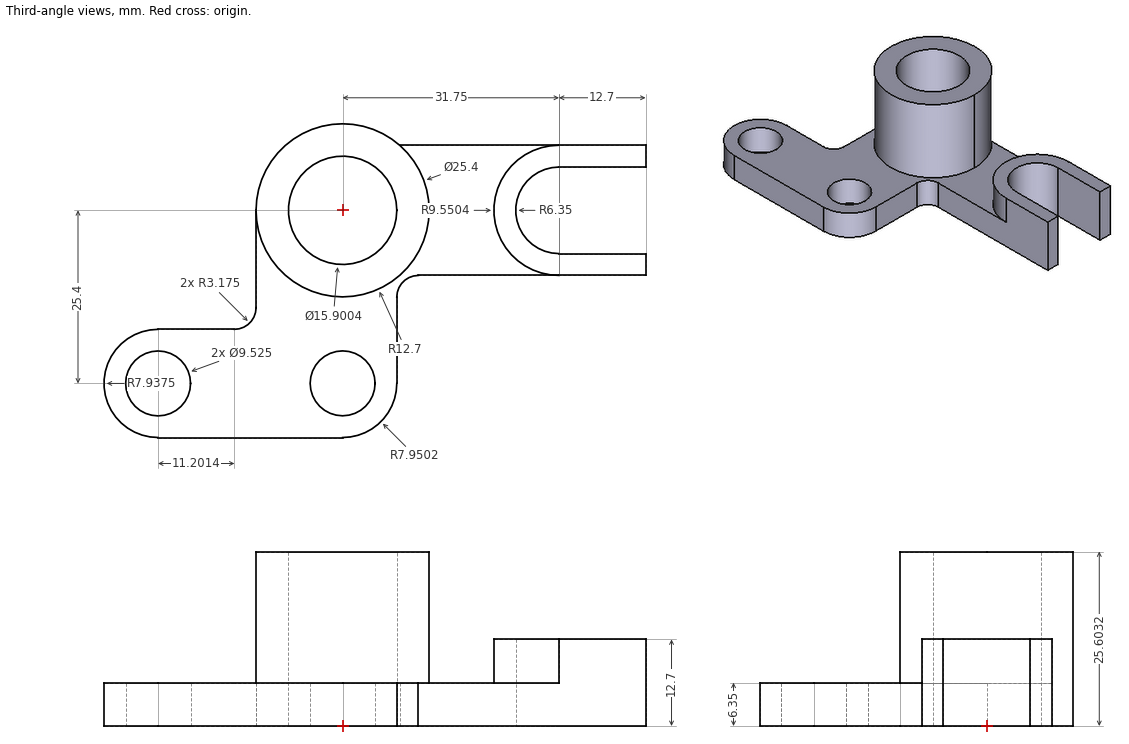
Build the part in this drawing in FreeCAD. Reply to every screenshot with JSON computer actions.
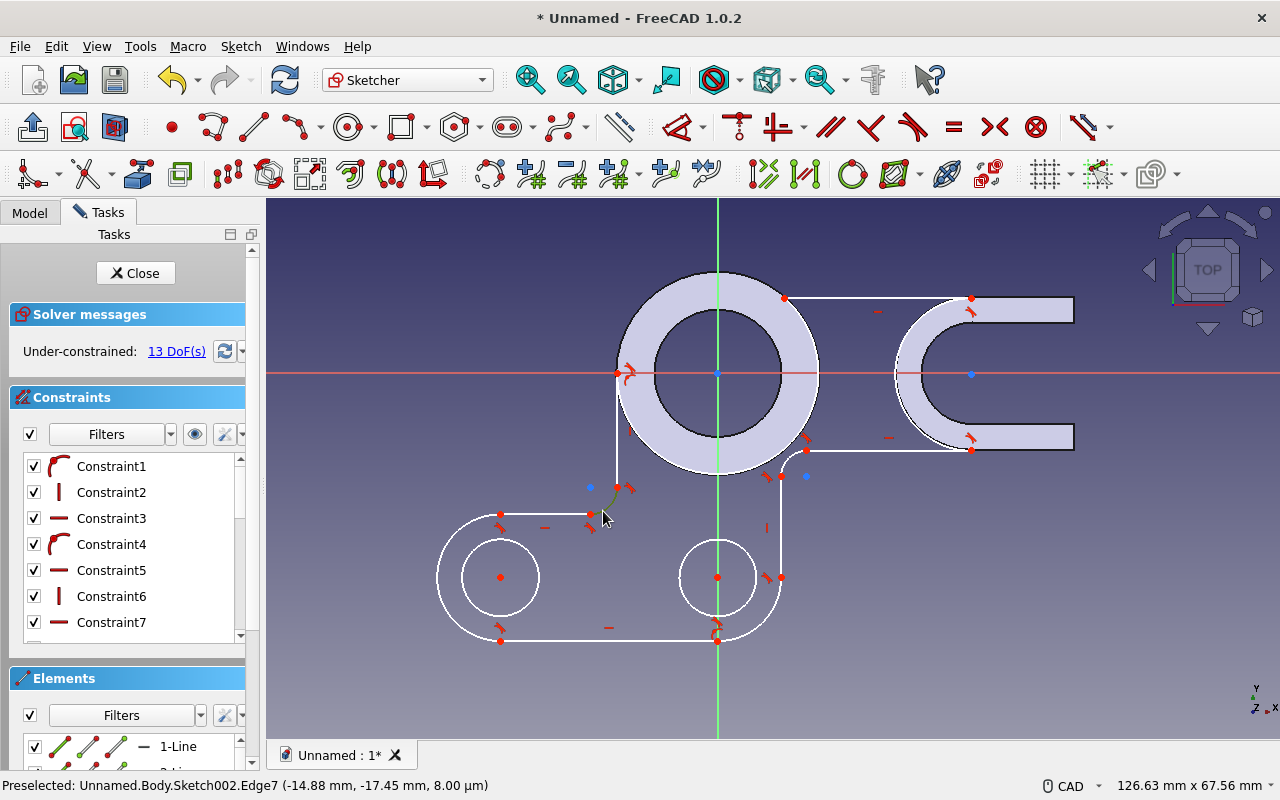
{"action": "scroll", "coordinate": [795, 454], "scroll_direction": "up", "scroll_amount": 2}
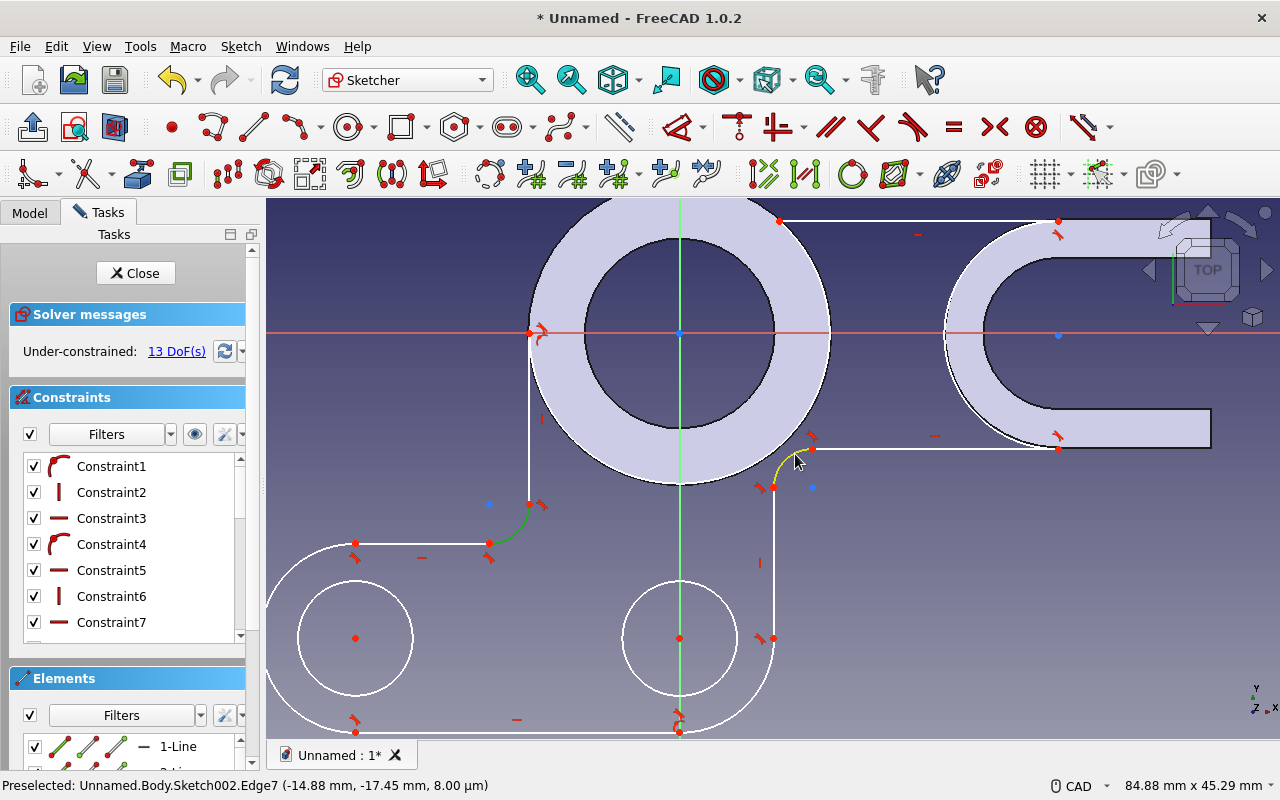
{"action": "left_click", "coordinate": [795, 453]}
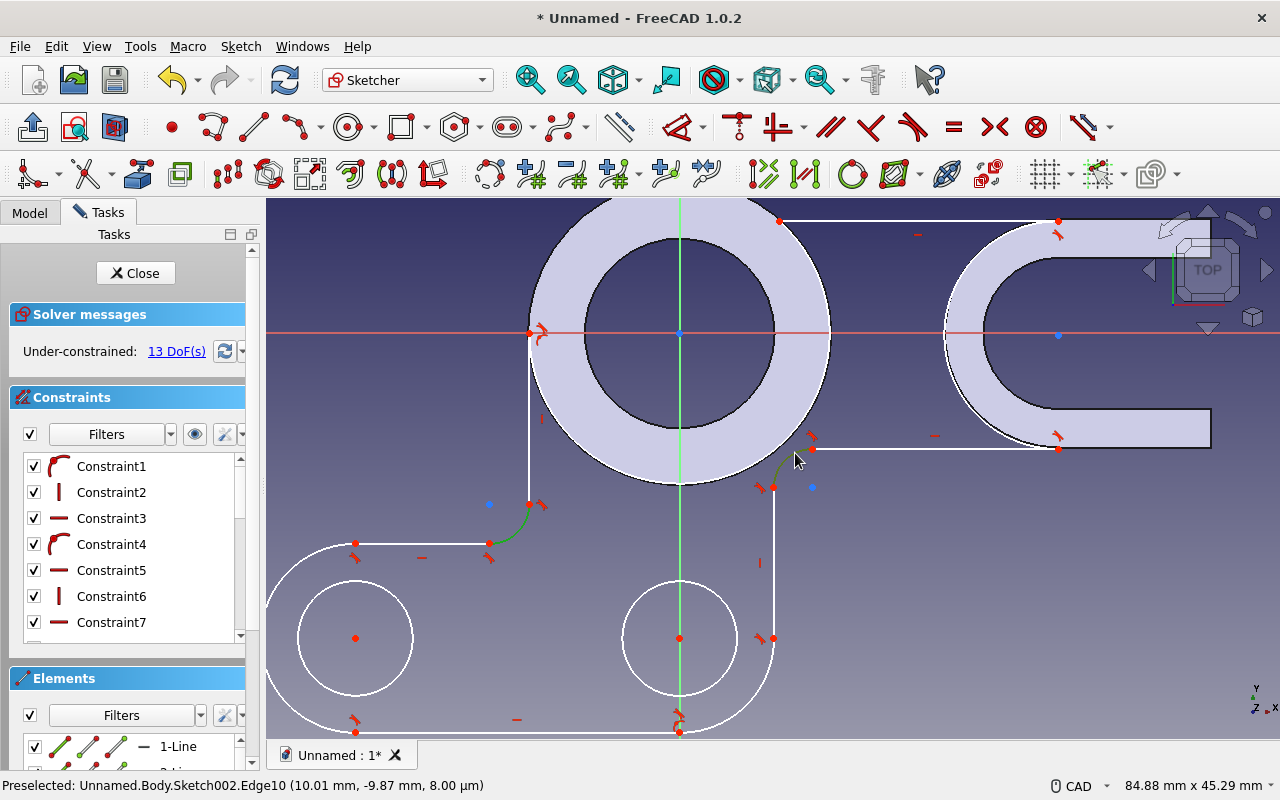
{"action": "left_click", "coordinate": [954, 128]}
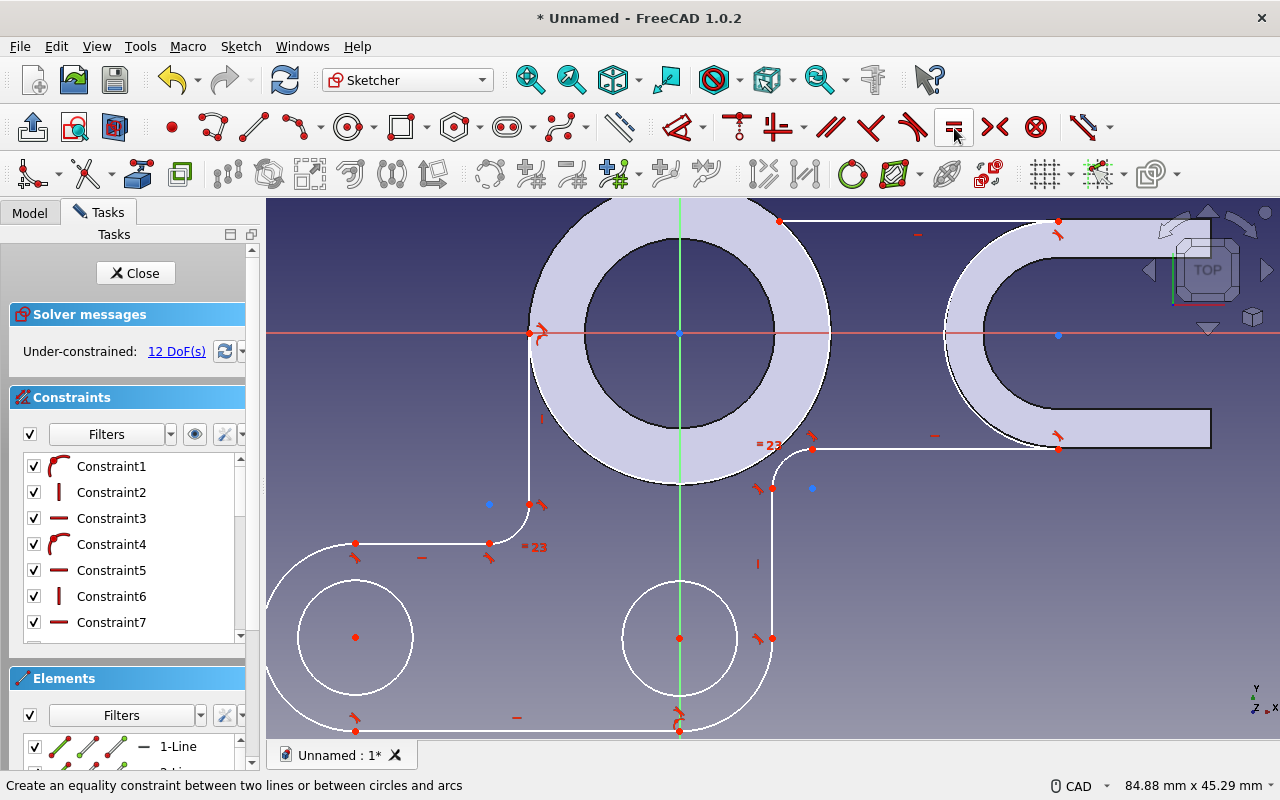
{"action": "left_click", "coordinate": [396, 597]}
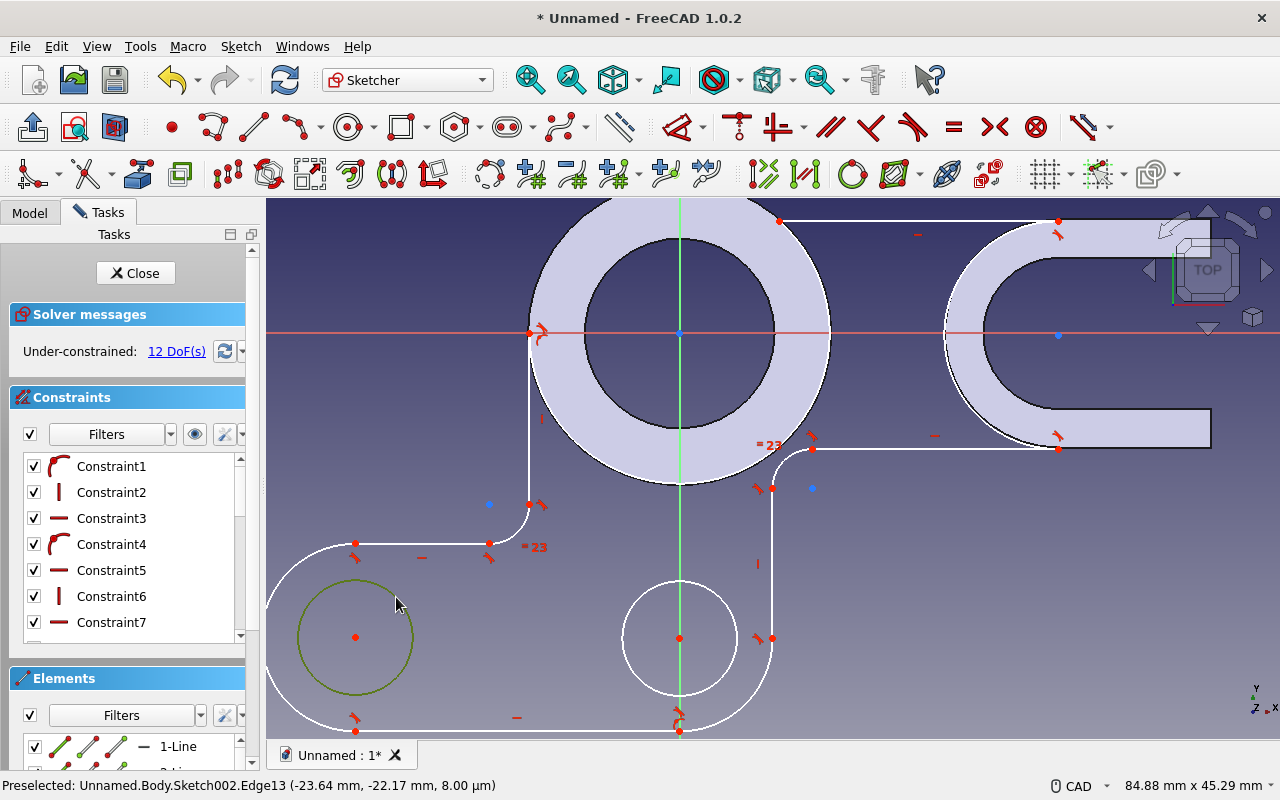
{"action": "left_click", "coordinate": [720, 598]}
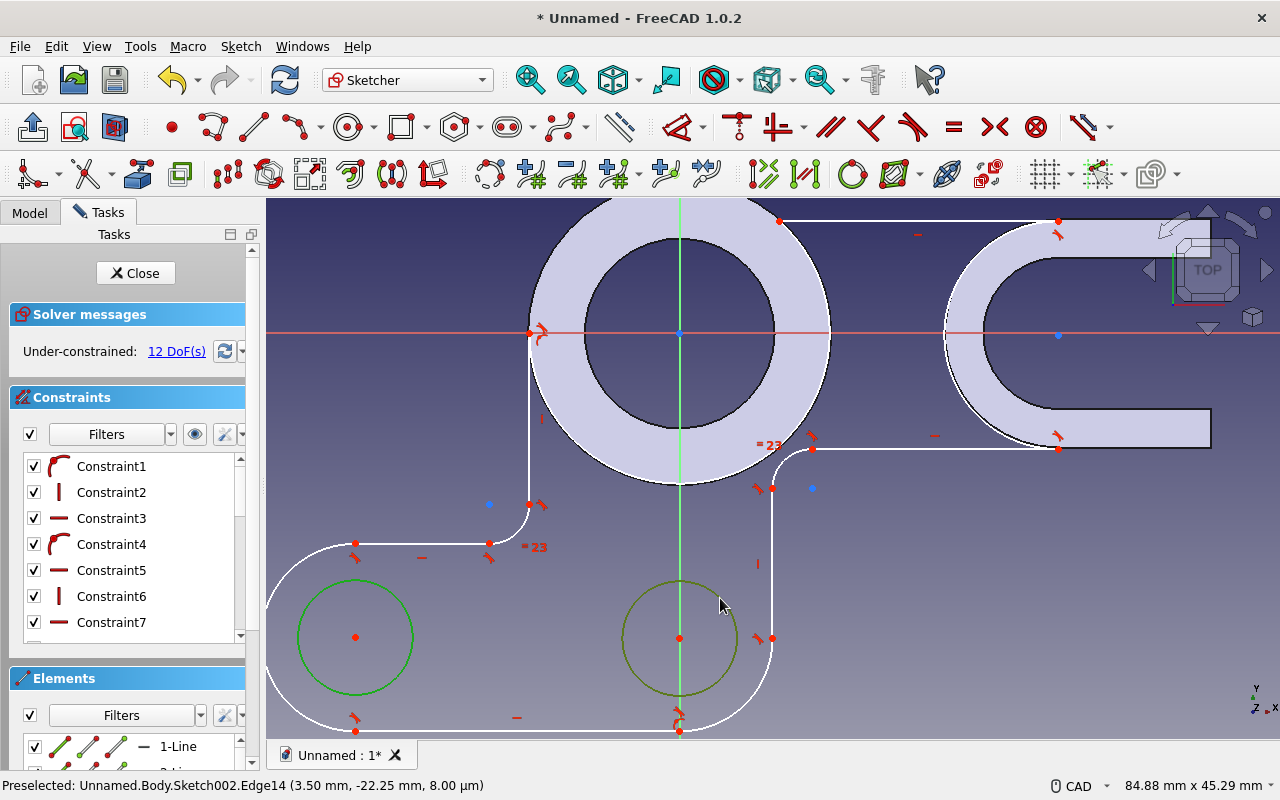
{"action": "left_click", "coordinate": [954, 128]}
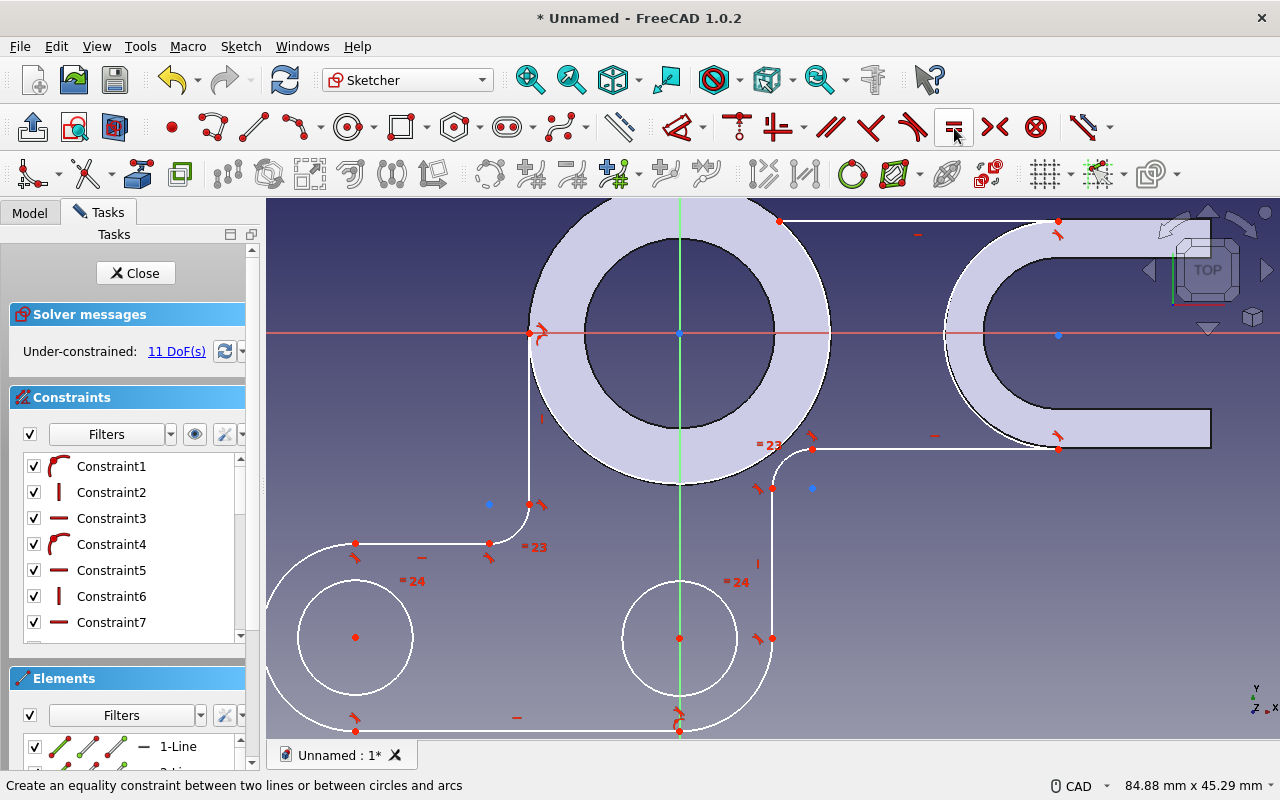
{"action": "left_click", "coordinate": [1058, 335]}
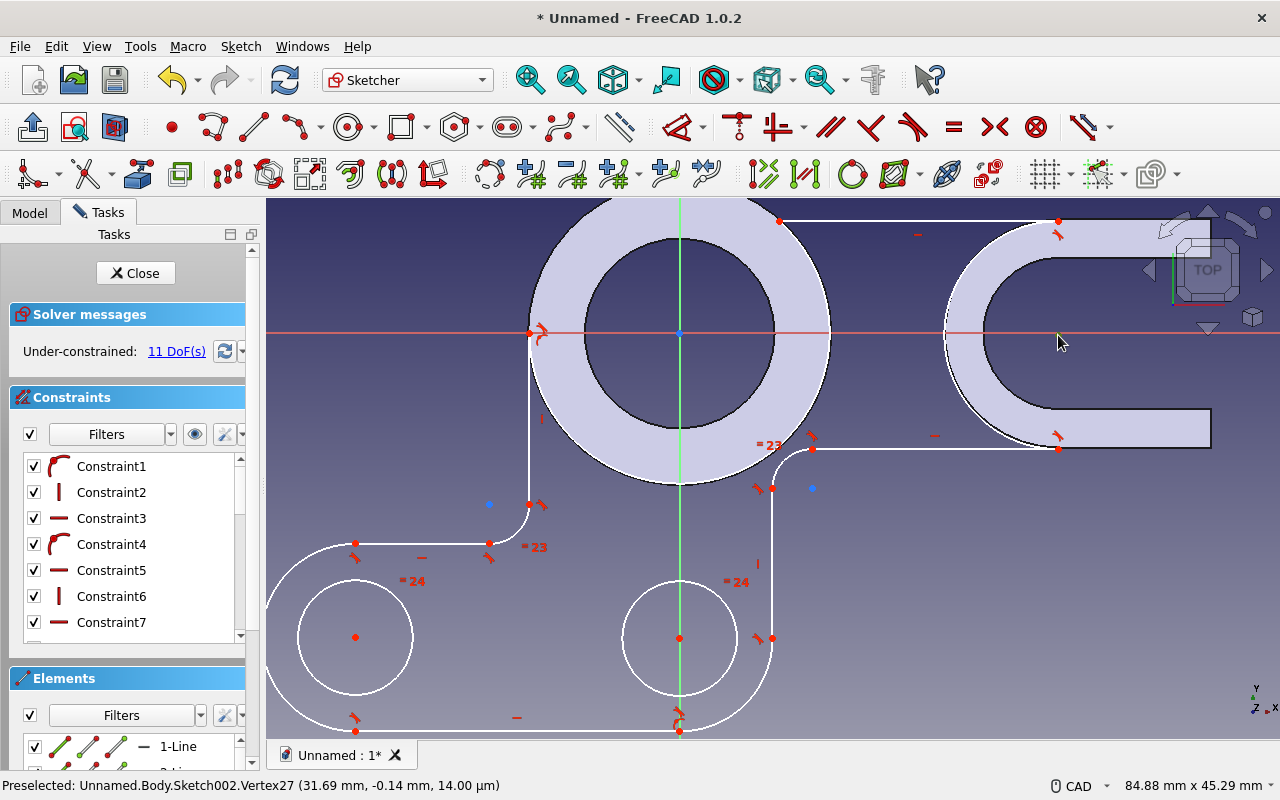
{"action": "left_click", "coordinate": [353, 333]}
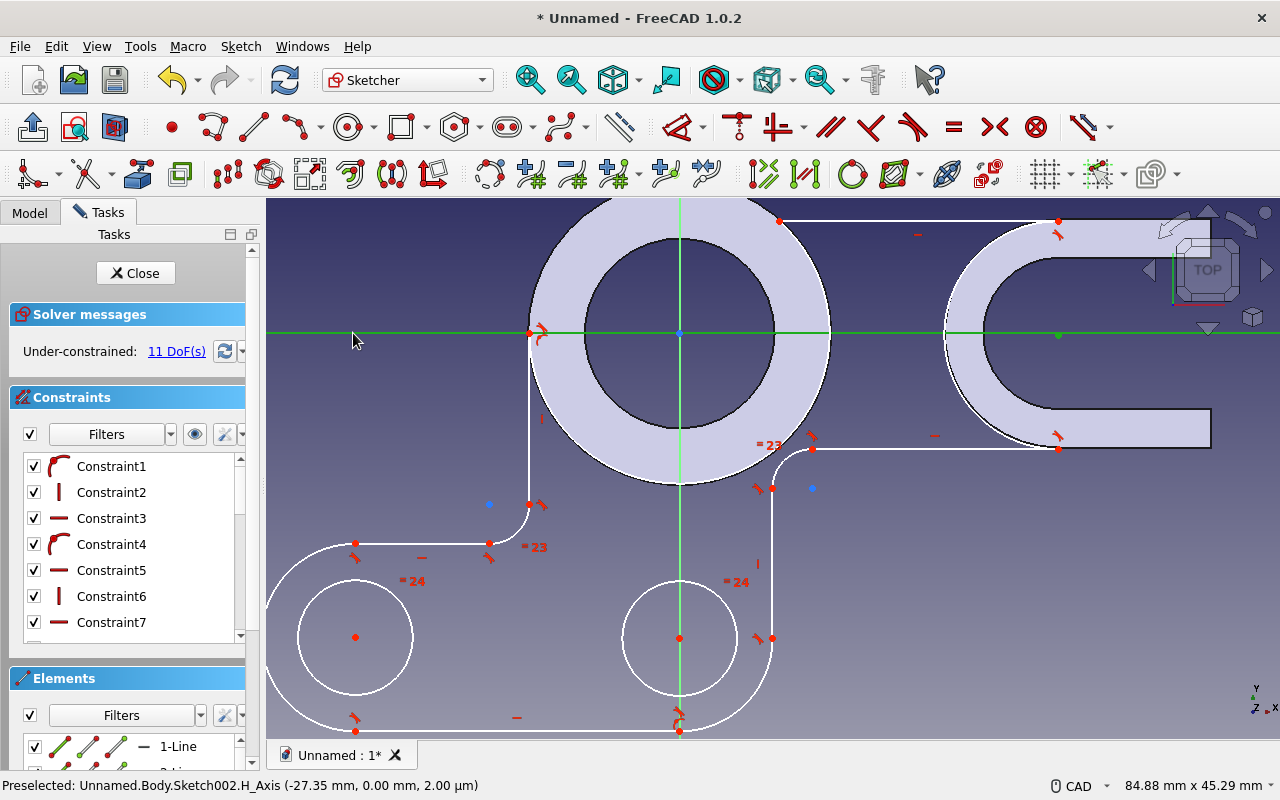
{"action": "left_click", "coordinate": [737, 128]}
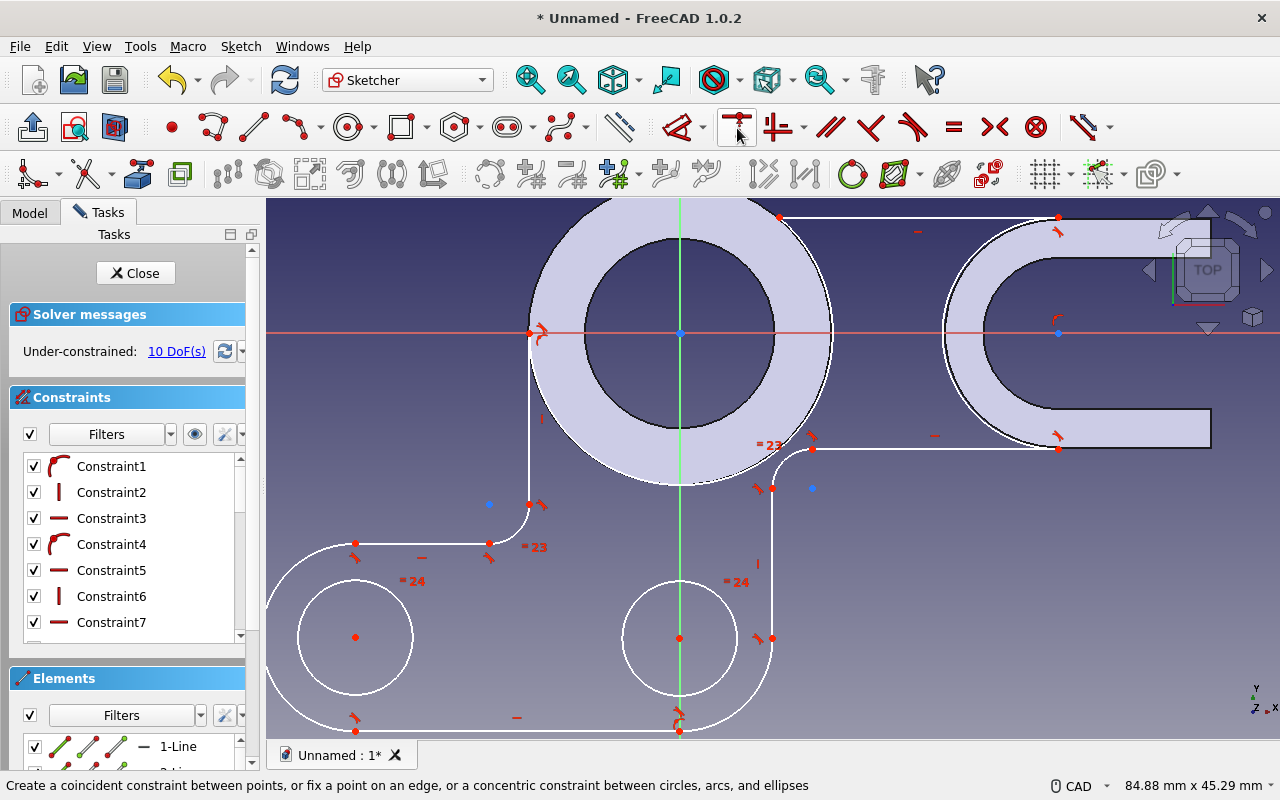
{"action": "left_click", "coordinate": [681, 333]}